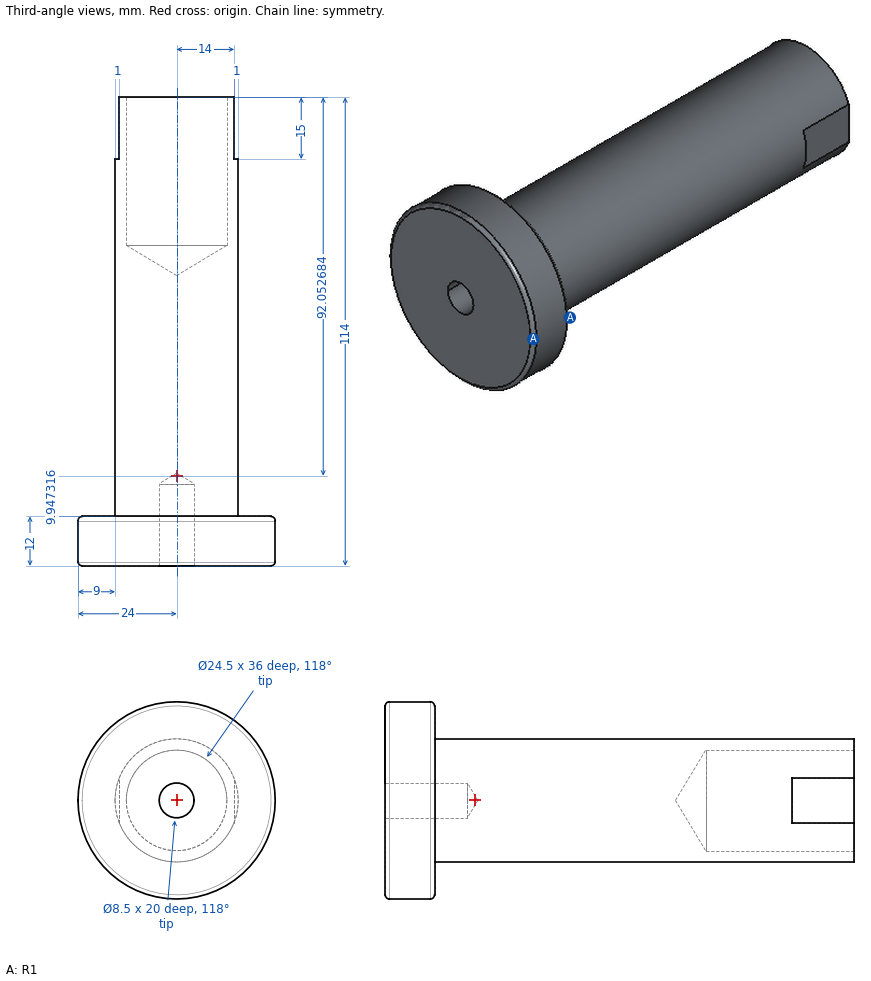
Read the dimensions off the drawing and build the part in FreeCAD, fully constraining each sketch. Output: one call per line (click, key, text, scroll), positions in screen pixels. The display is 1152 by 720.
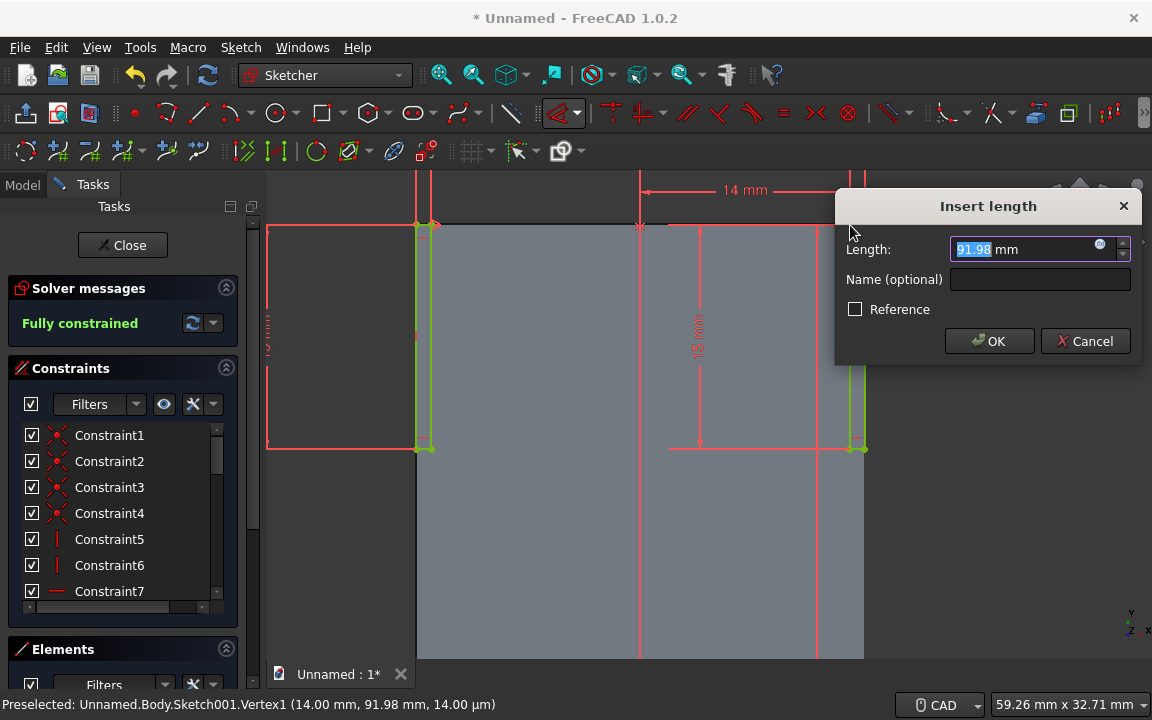
text(92.052684)
key(Return)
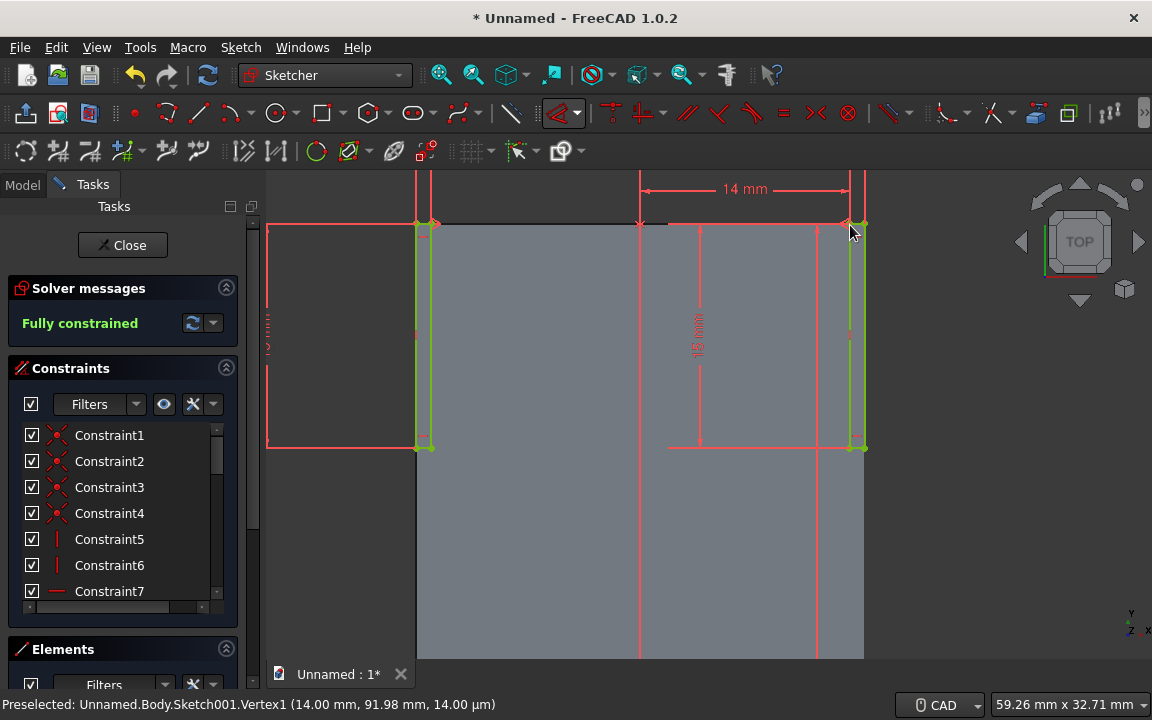
click(123, 245)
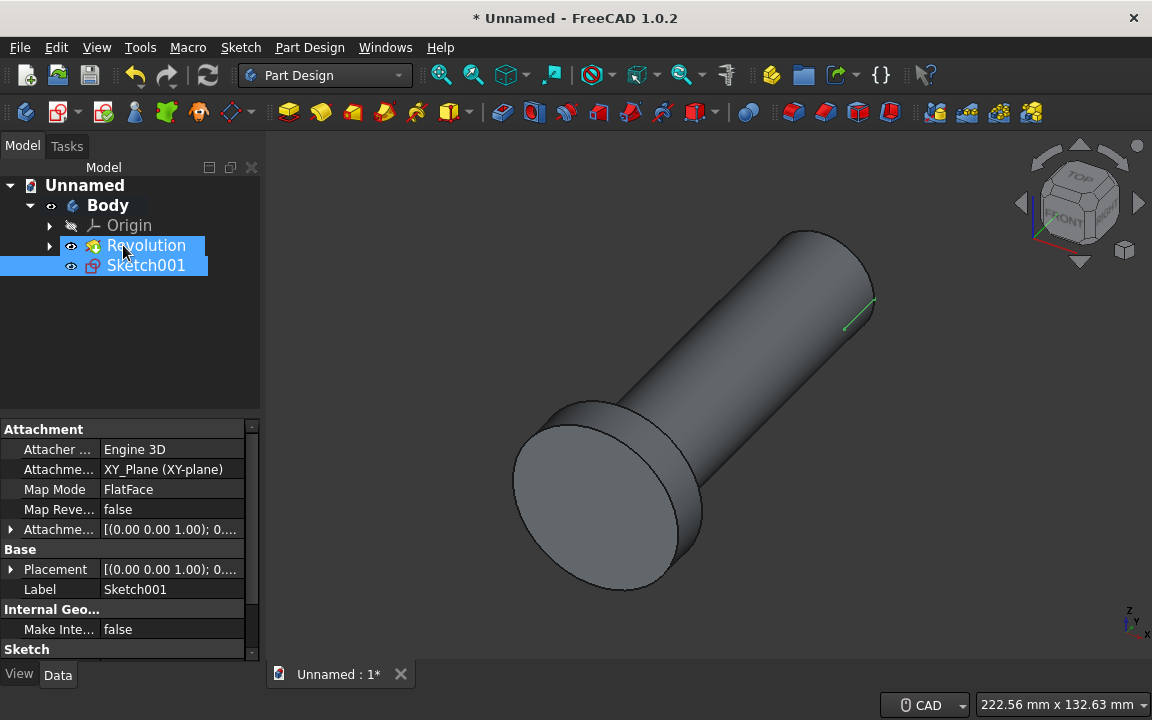
click(504, 112)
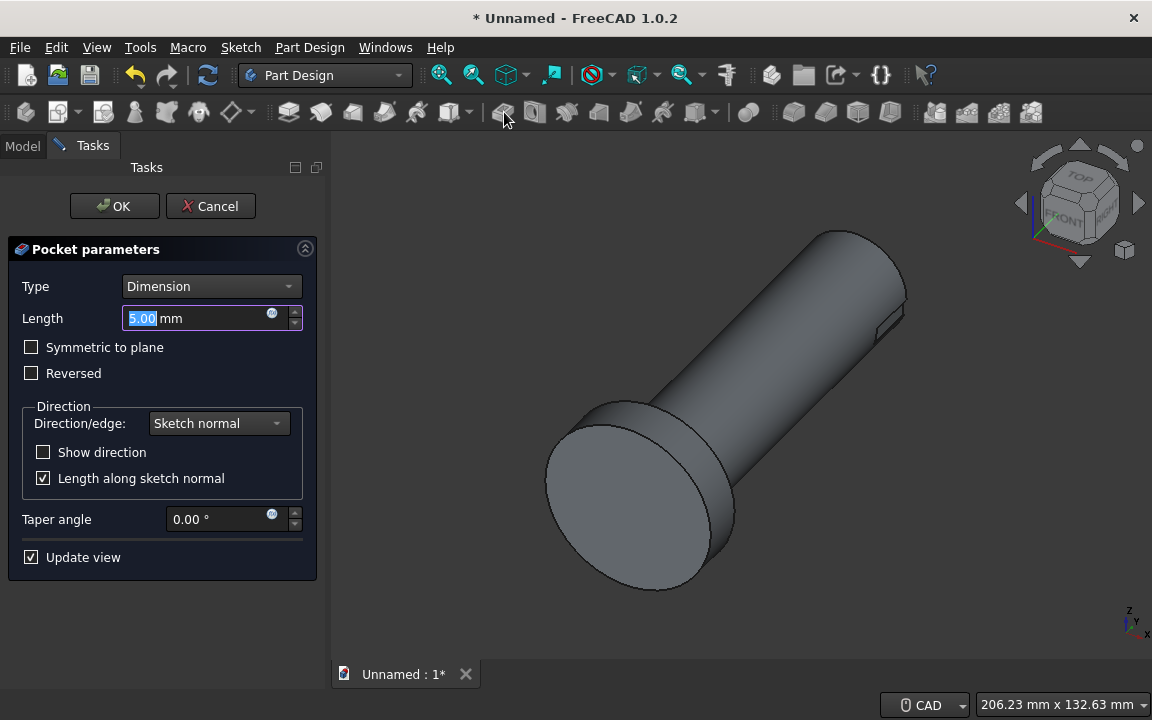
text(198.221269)
key(Tab)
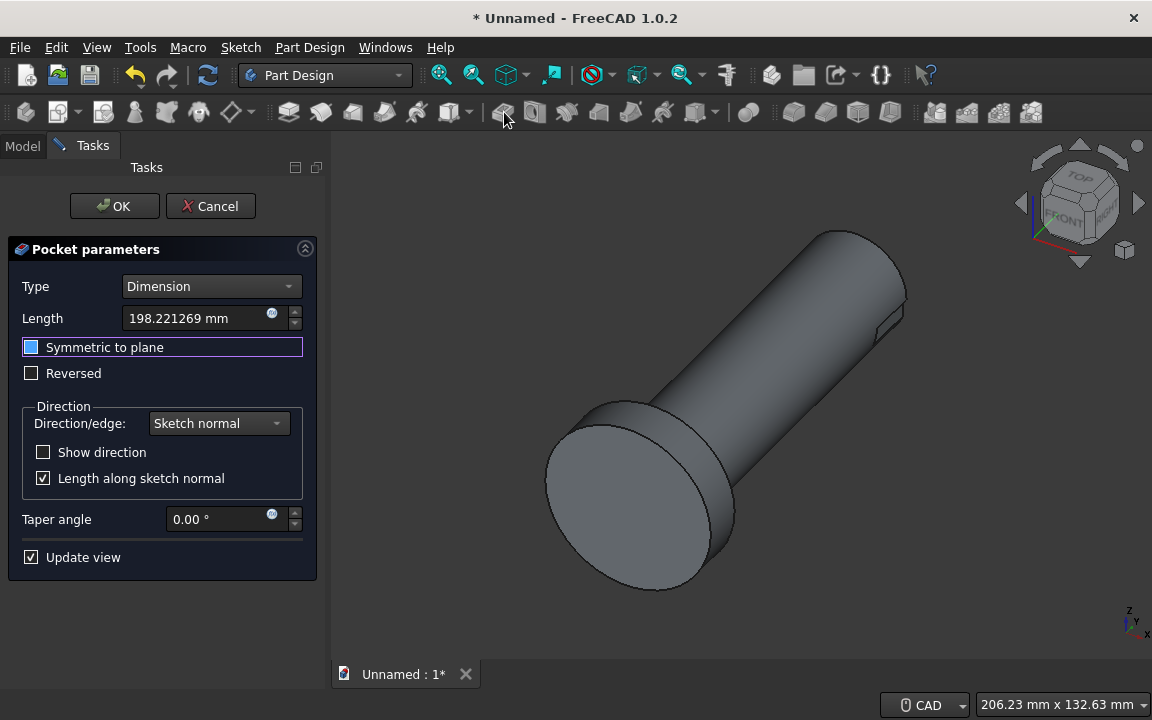
click(30, 347)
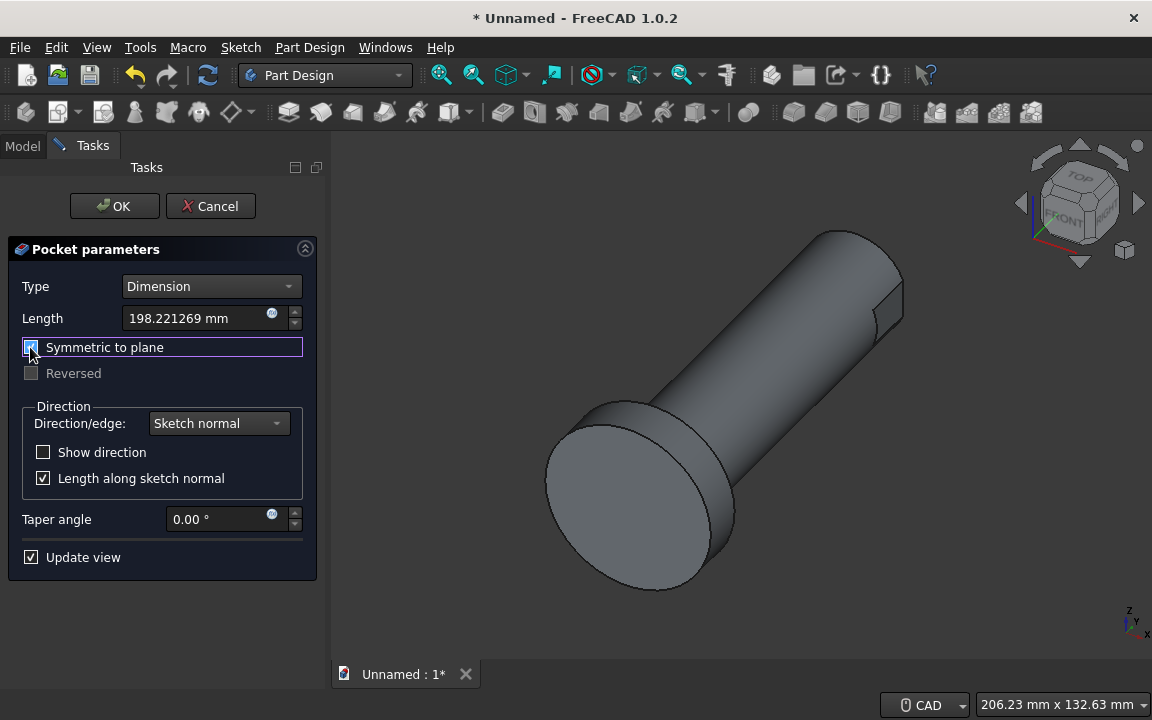
click(115, 206)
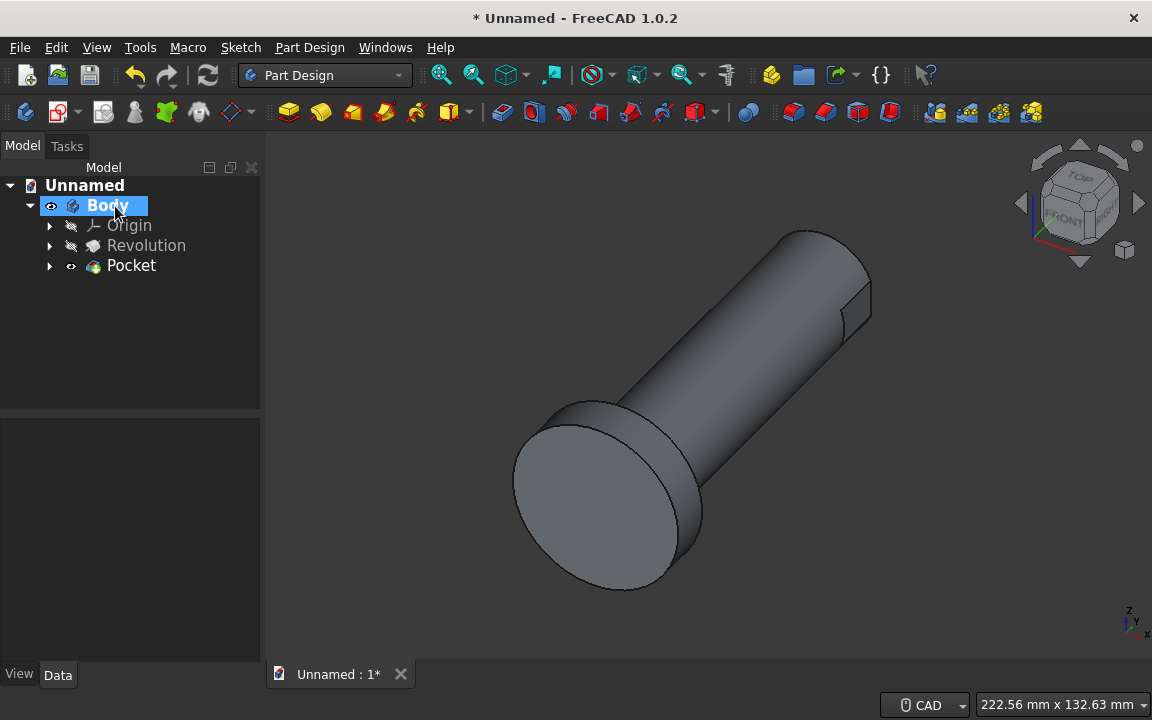
click(678, 534)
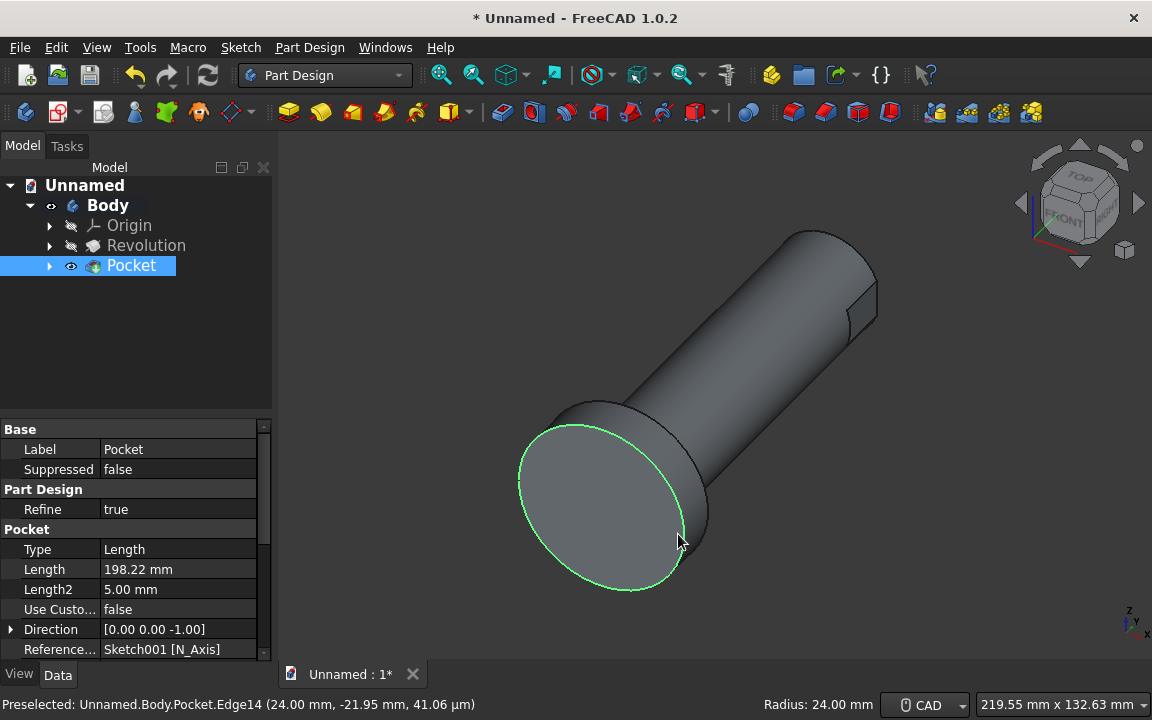
key(0)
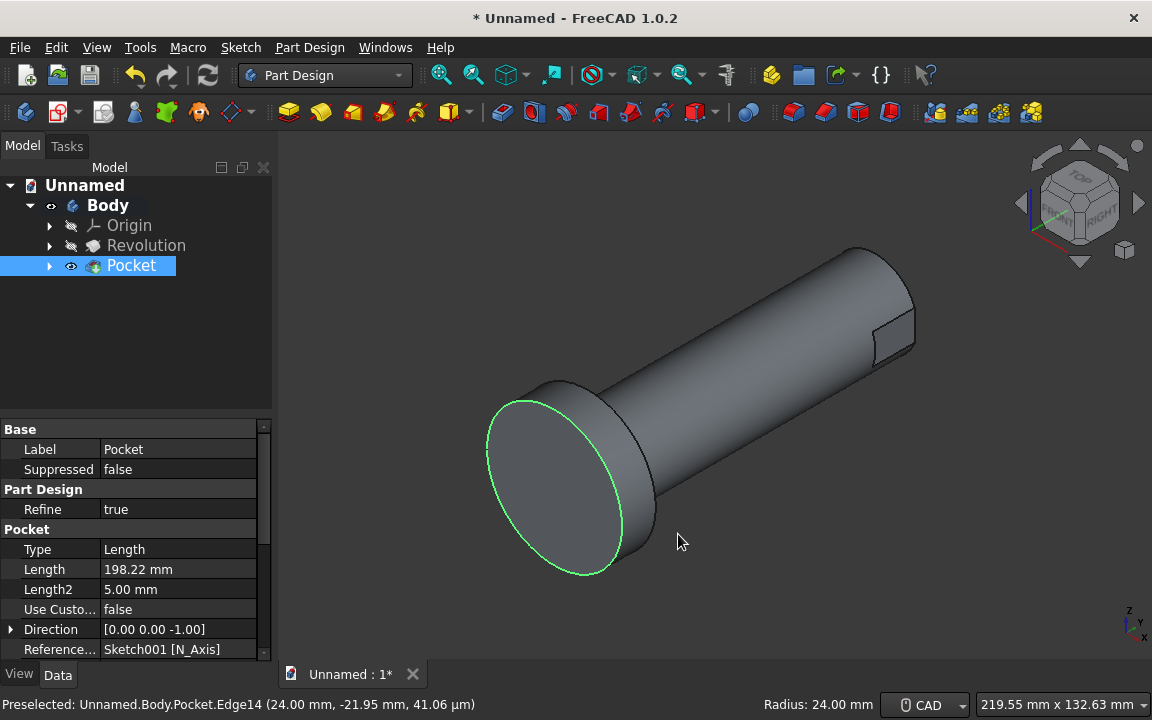
key(2)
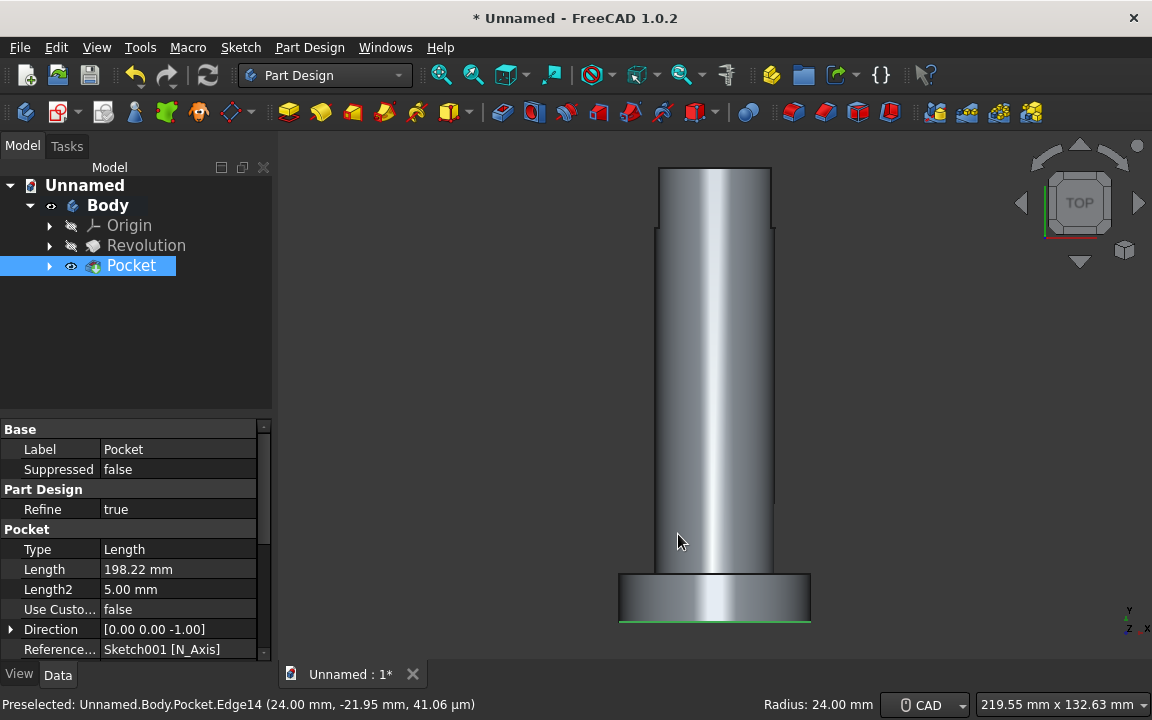
click(792, 573, ctrl)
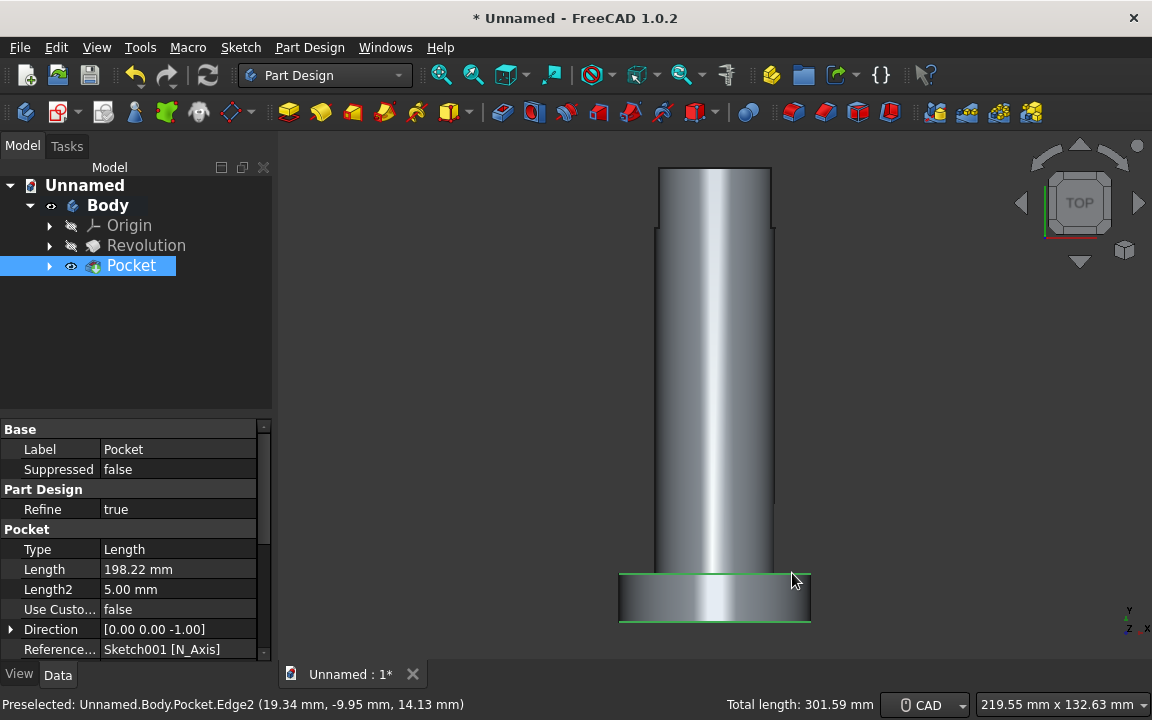
click(794, 112)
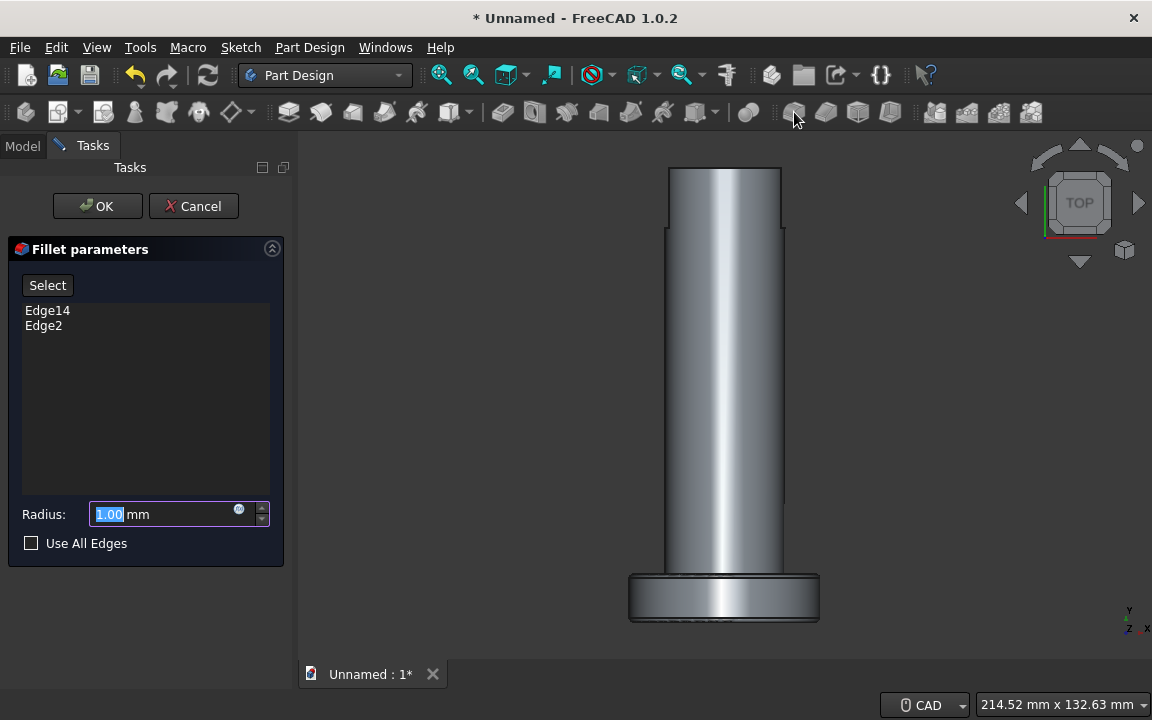
text(1)
key(Tab)